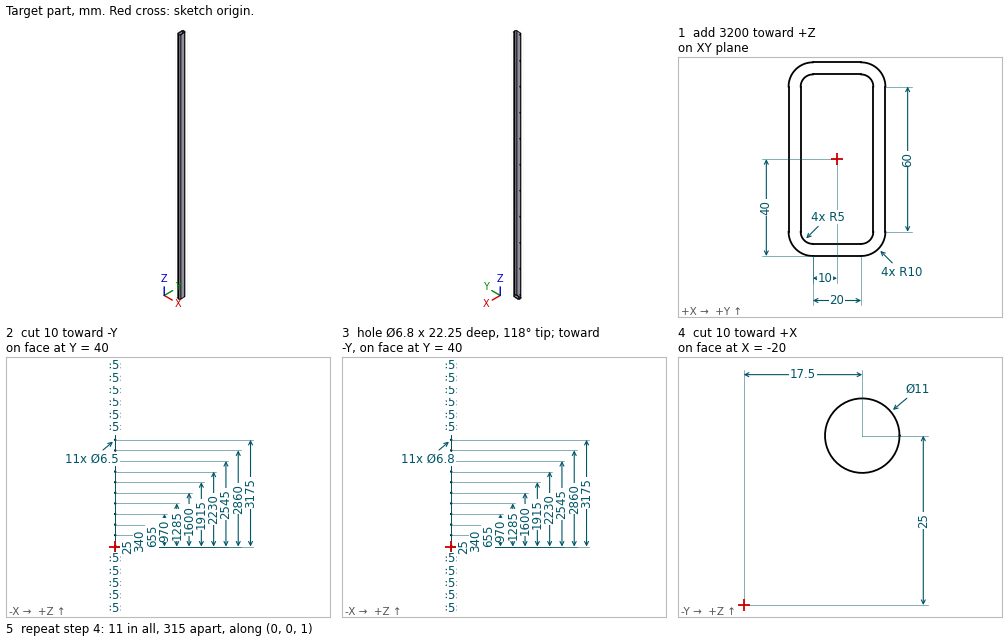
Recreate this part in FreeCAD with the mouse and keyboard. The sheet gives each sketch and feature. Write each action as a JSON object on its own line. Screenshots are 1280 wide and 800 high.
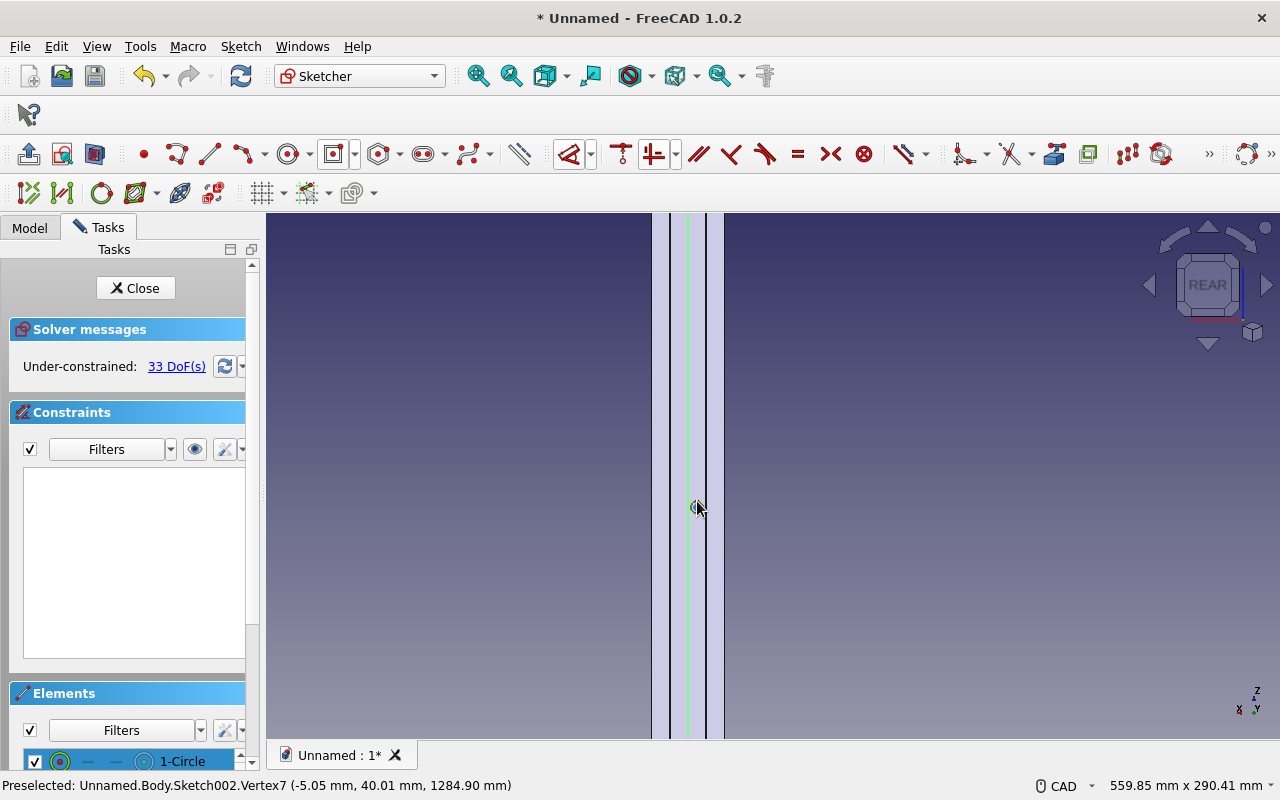
{"action": "scroll", "coordinate": [705, 510], "scroll_direction": "down", "scroll_amount": 14}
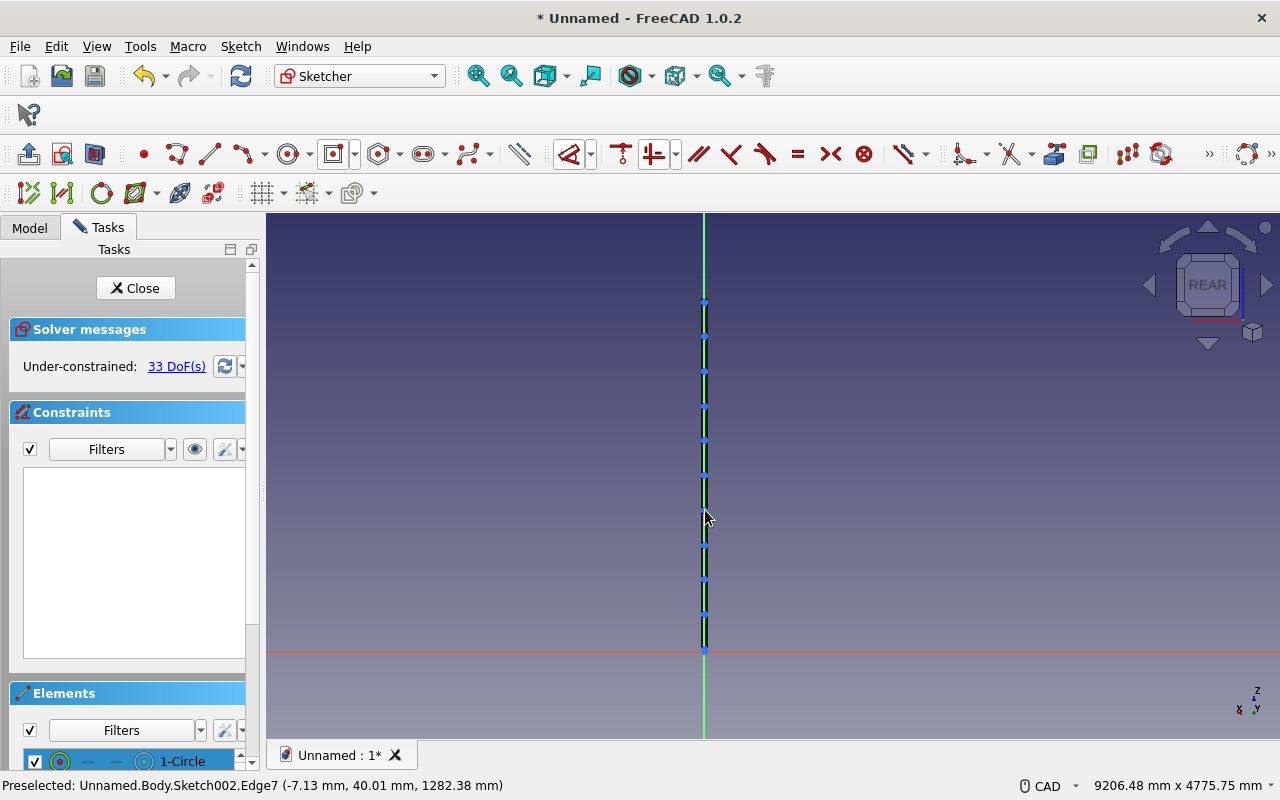
{"action": "scroll", "coordinate": [705, 545], "scroll_direction": "up", "scroll_amount": 14}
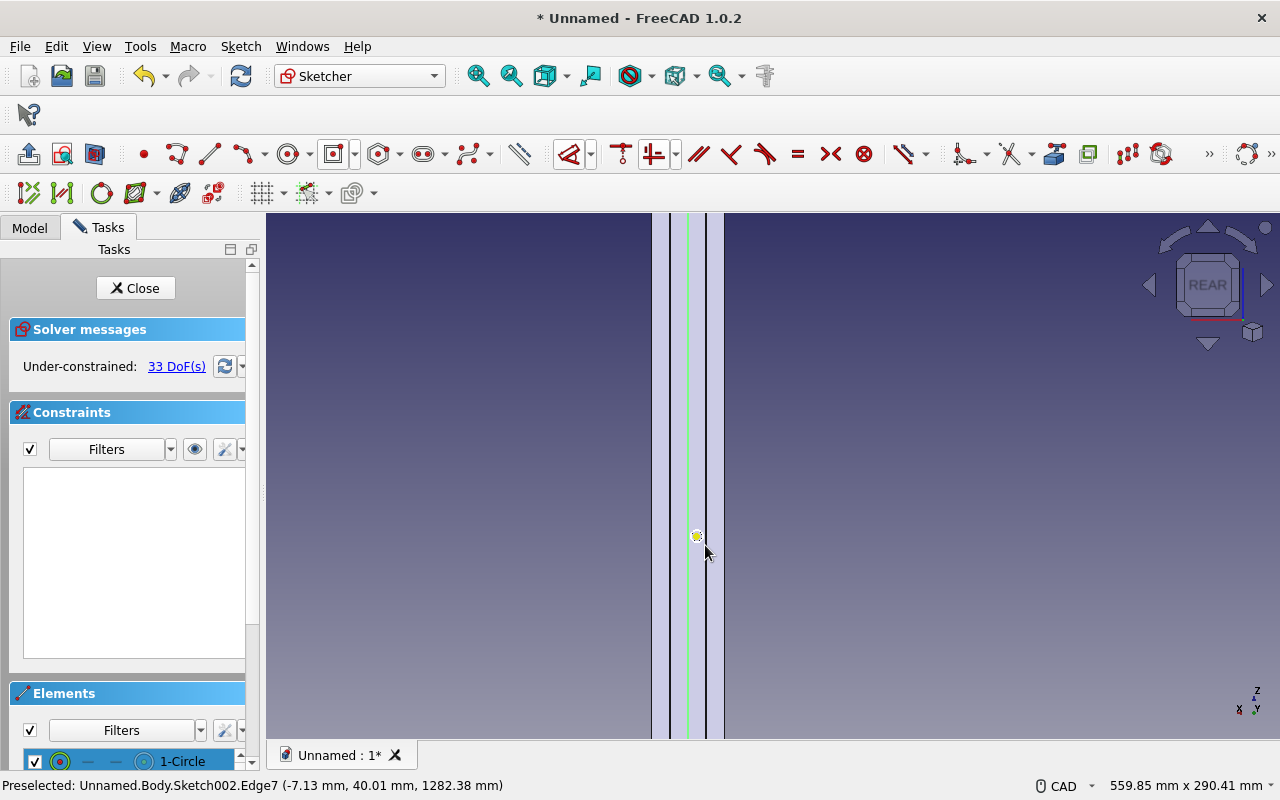
{"action": "left_click", "coordinate": [701, 541]}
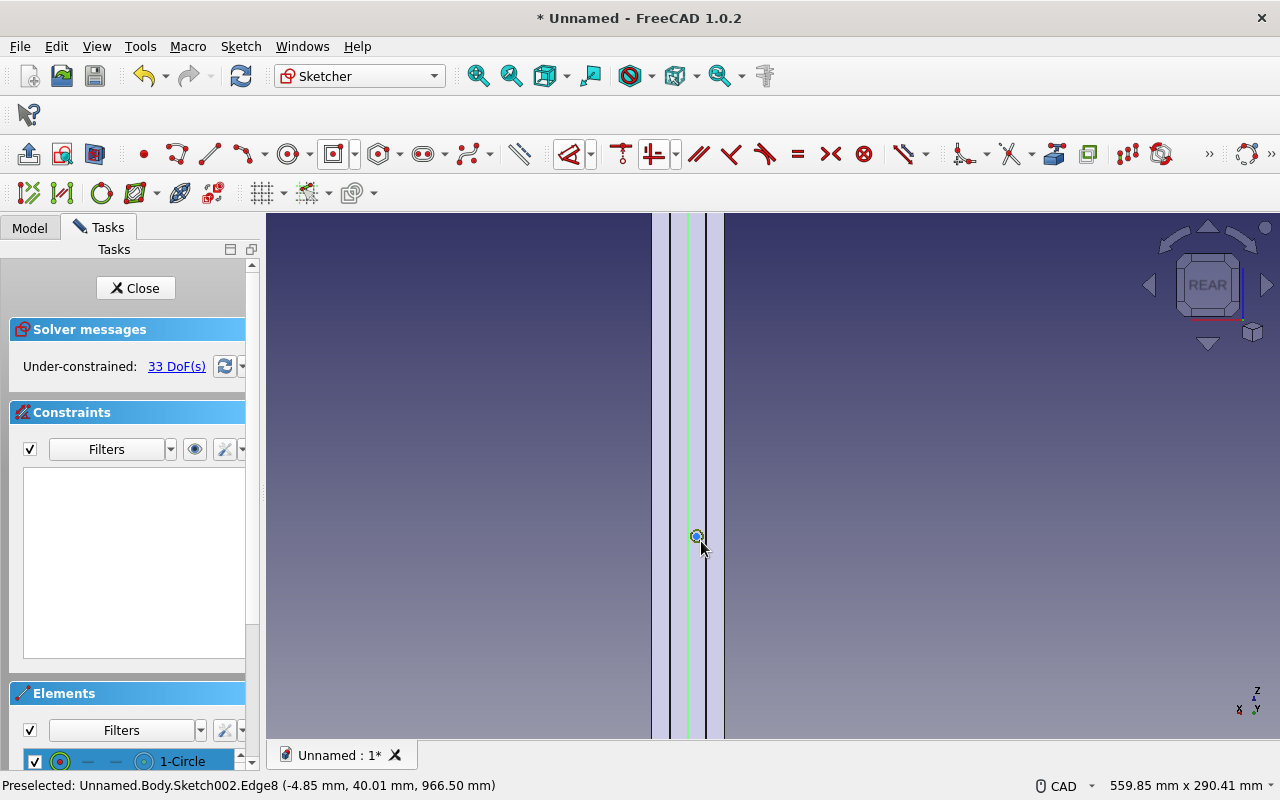
{"action": "scroll", "coordinate": [705, 545], "scroll_direction": "down", "scroll_amount": 14}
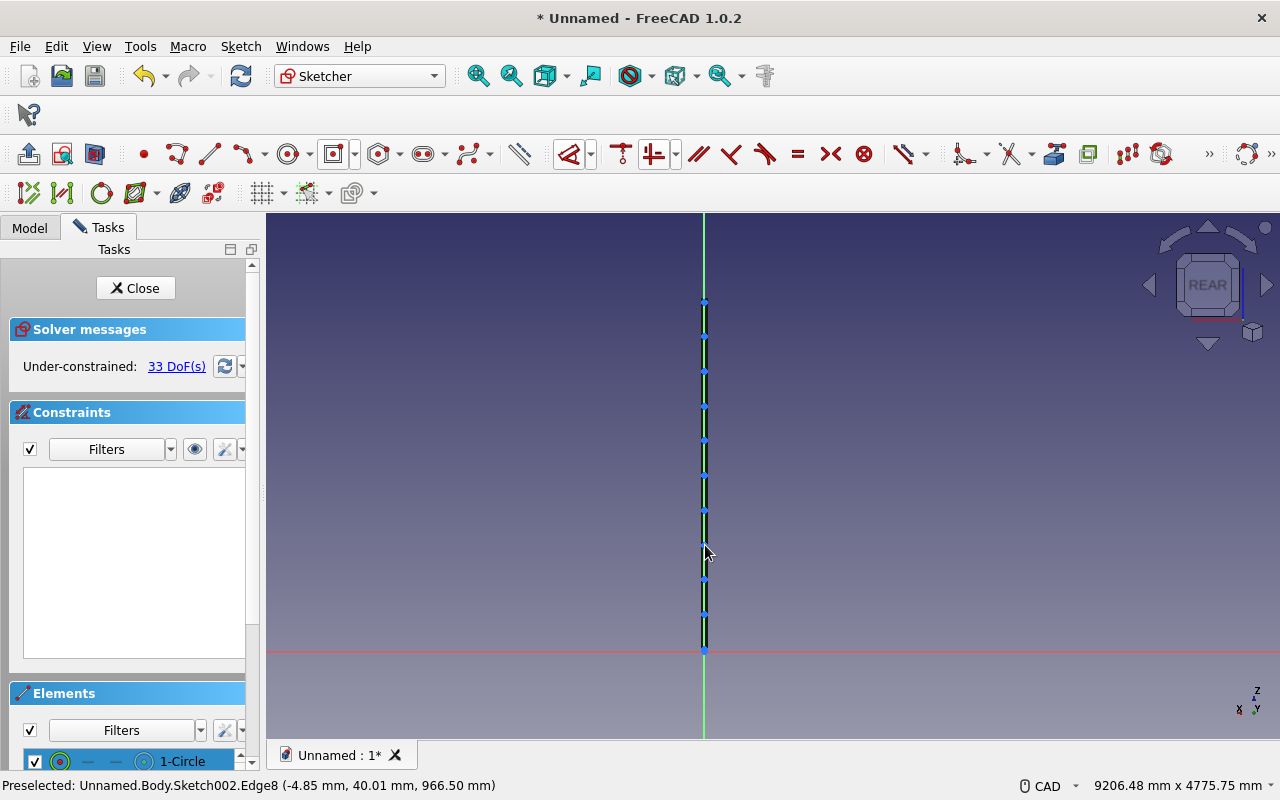
{"action": "scroll", "coordinate": [705, 580], "scroll_direction": "up", "scroll_amount": 14}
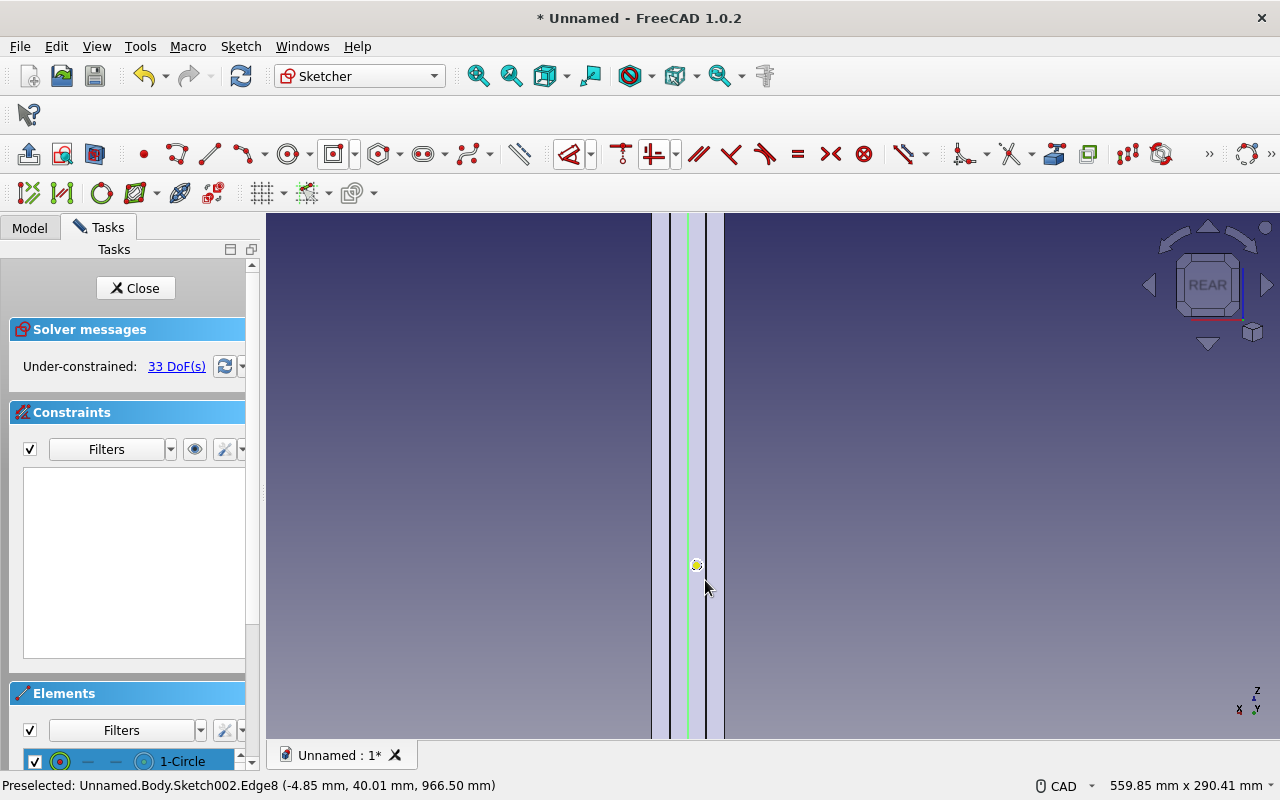
{"action": "left_click", "coordinate": [701, 570]}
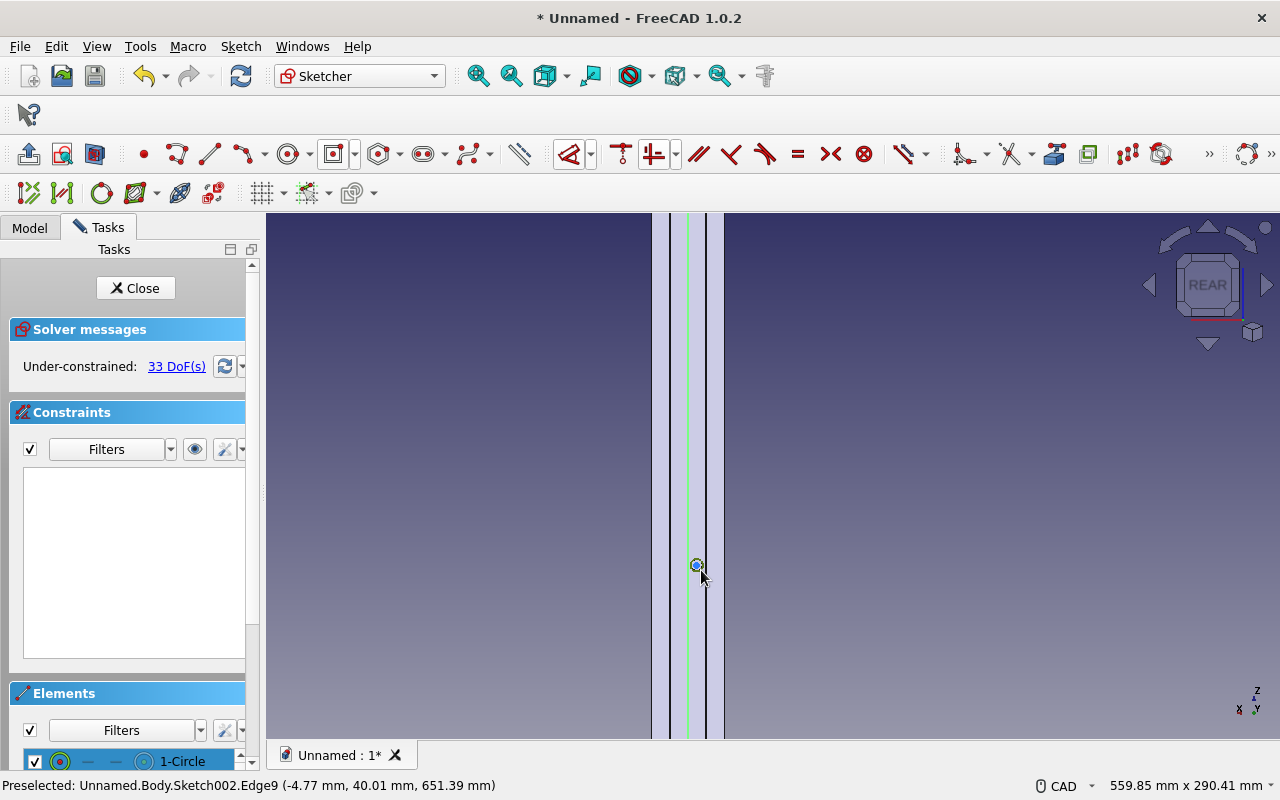
{"action": "scroll", "coordinate": [705, 580], "scroll_direction": "down", "scroll_amount": 14}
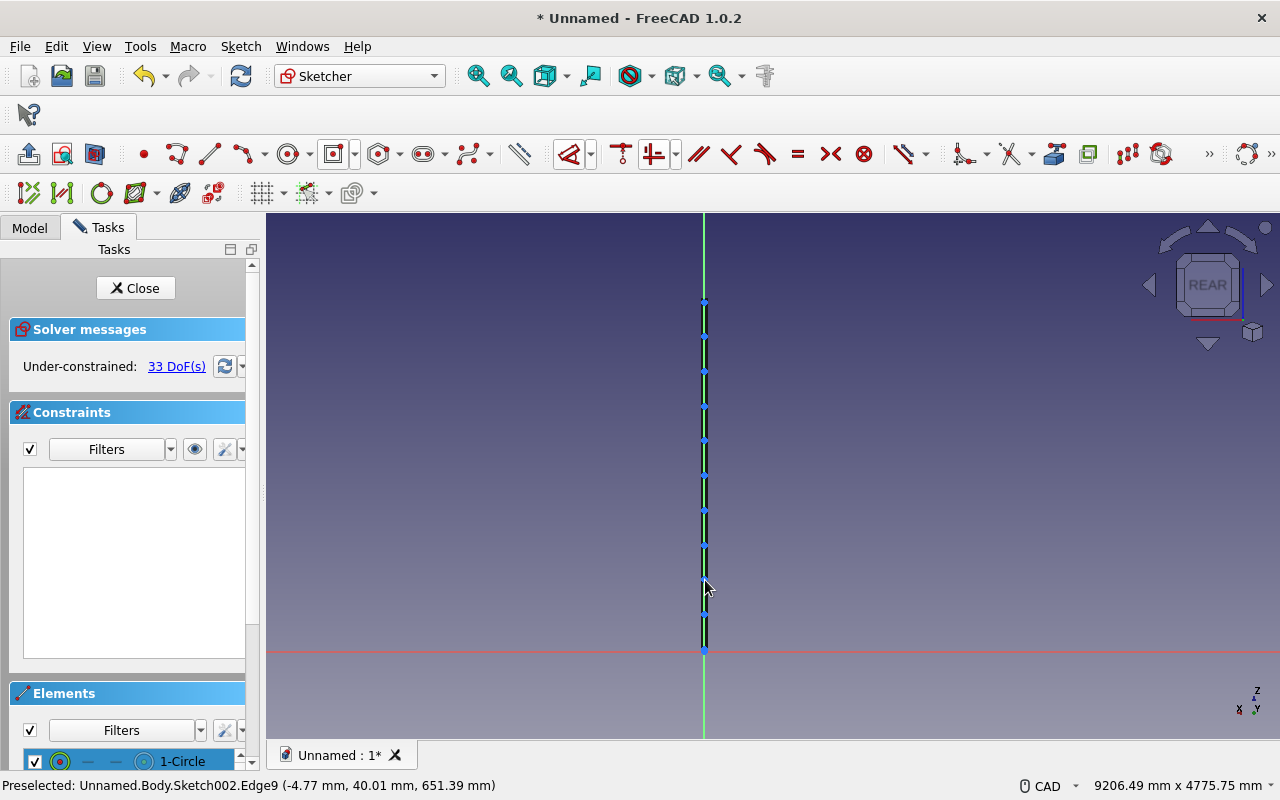
{"action": "scroll", "coordinate": [705, 614], "scroll_direction": "up", "scroll_amount": 14}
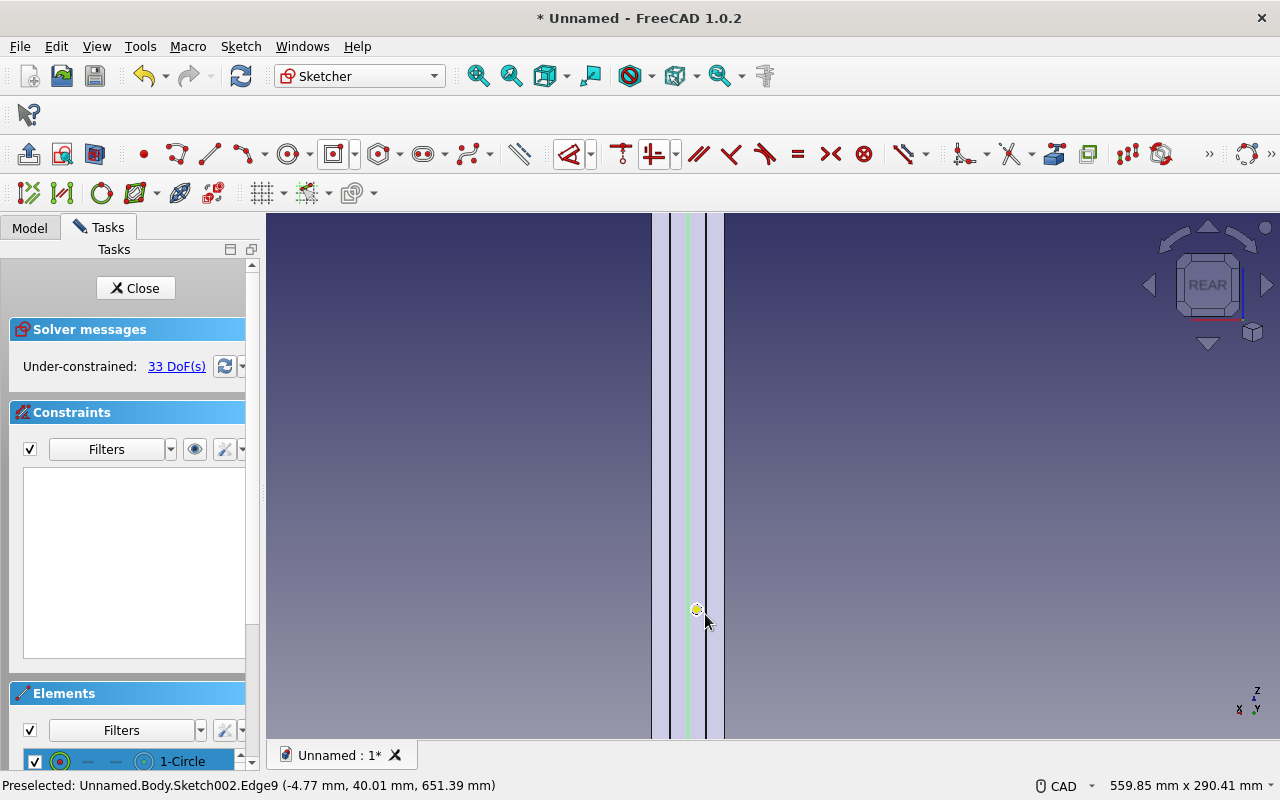
{"action": "left_click", "coordinate": [697, 603]}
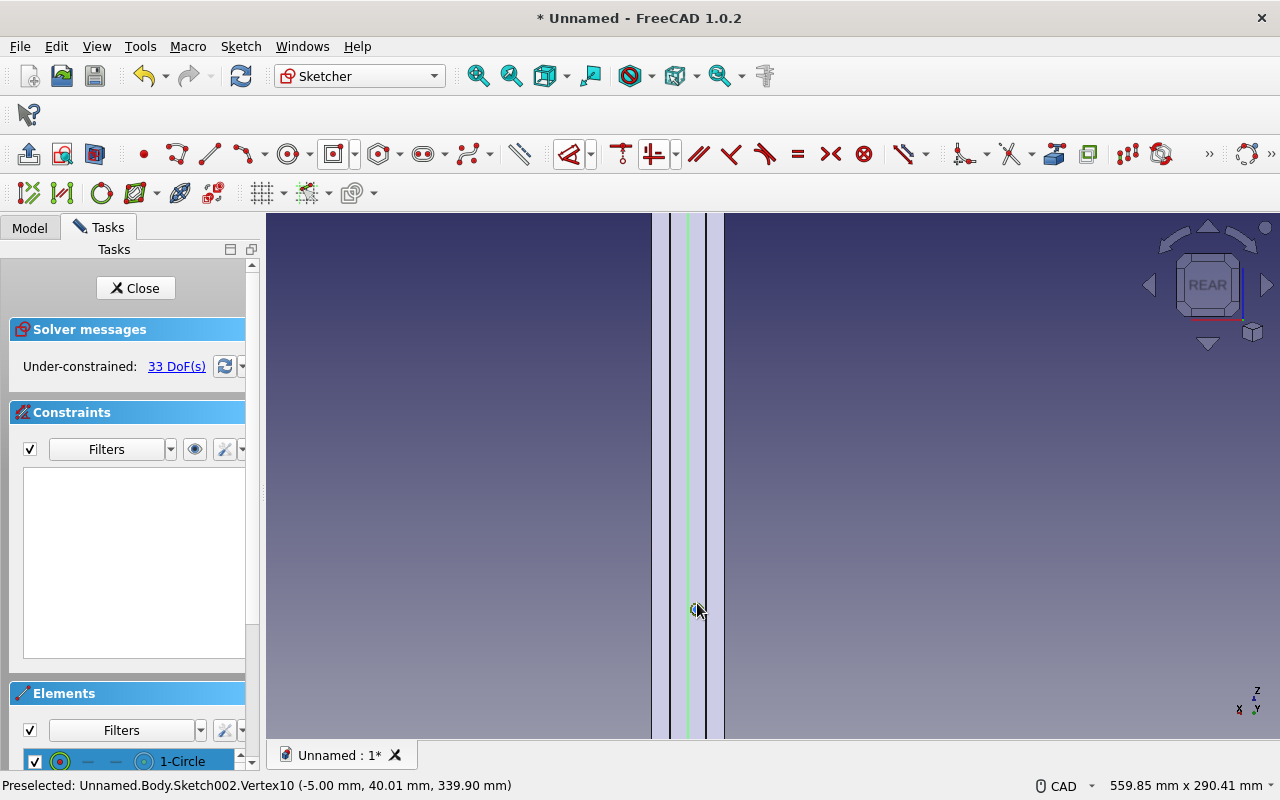
{"action": "scroll", "coordinate": [705, 614], "scroll_direction": "down", "scroll_amount": 14}